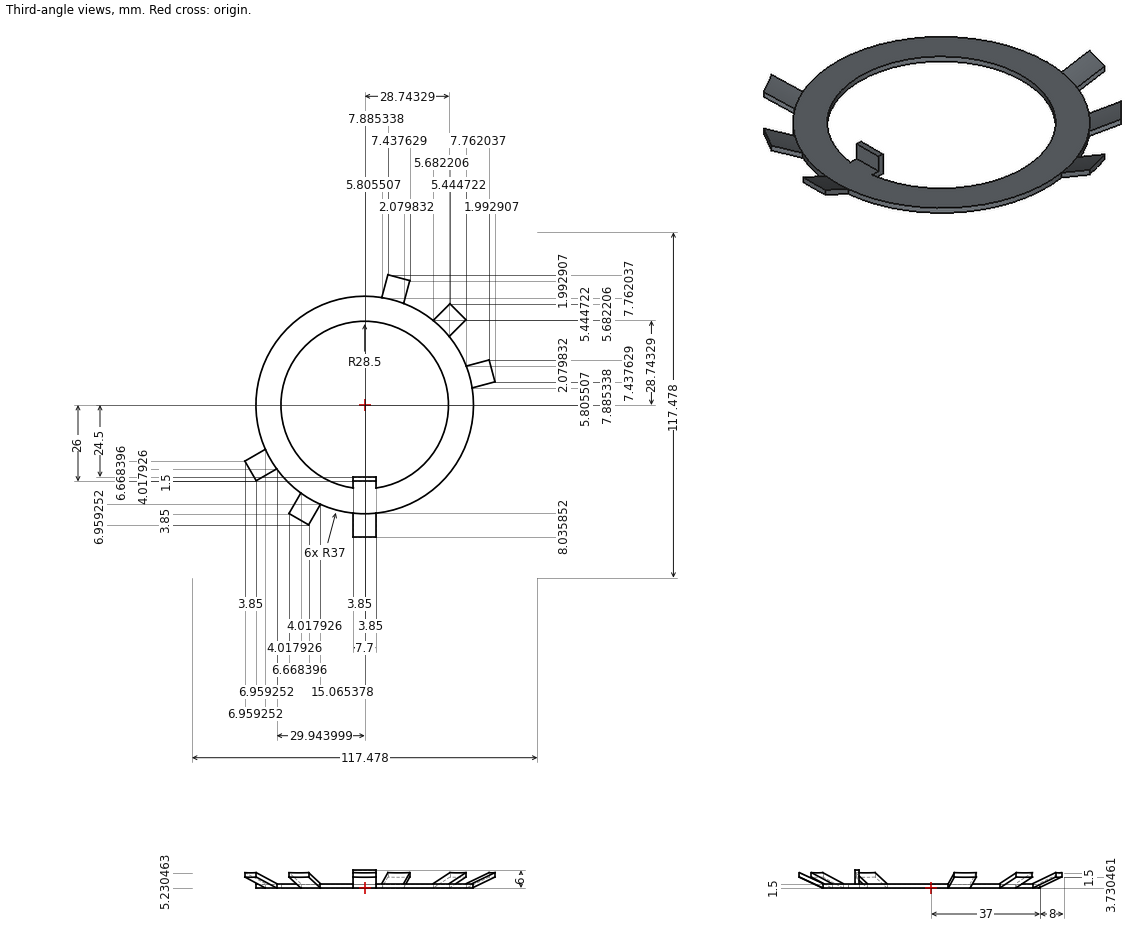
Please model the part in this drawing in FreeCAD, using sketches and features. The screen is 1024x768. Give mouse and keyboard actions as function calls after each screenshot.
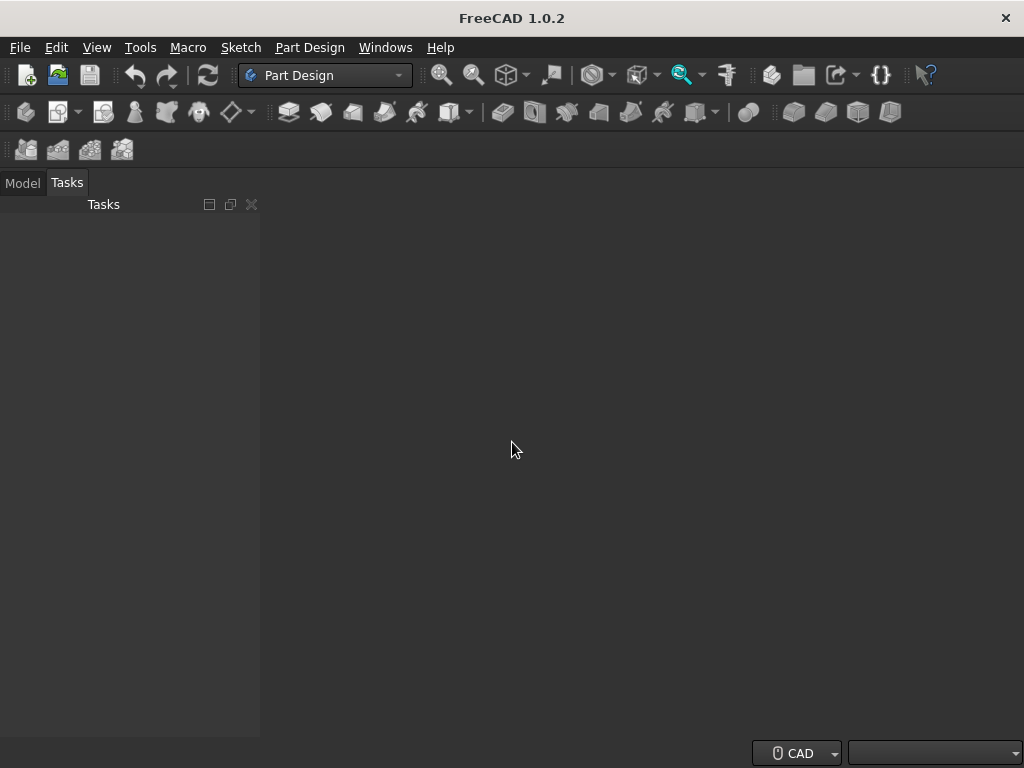
click(26, 76)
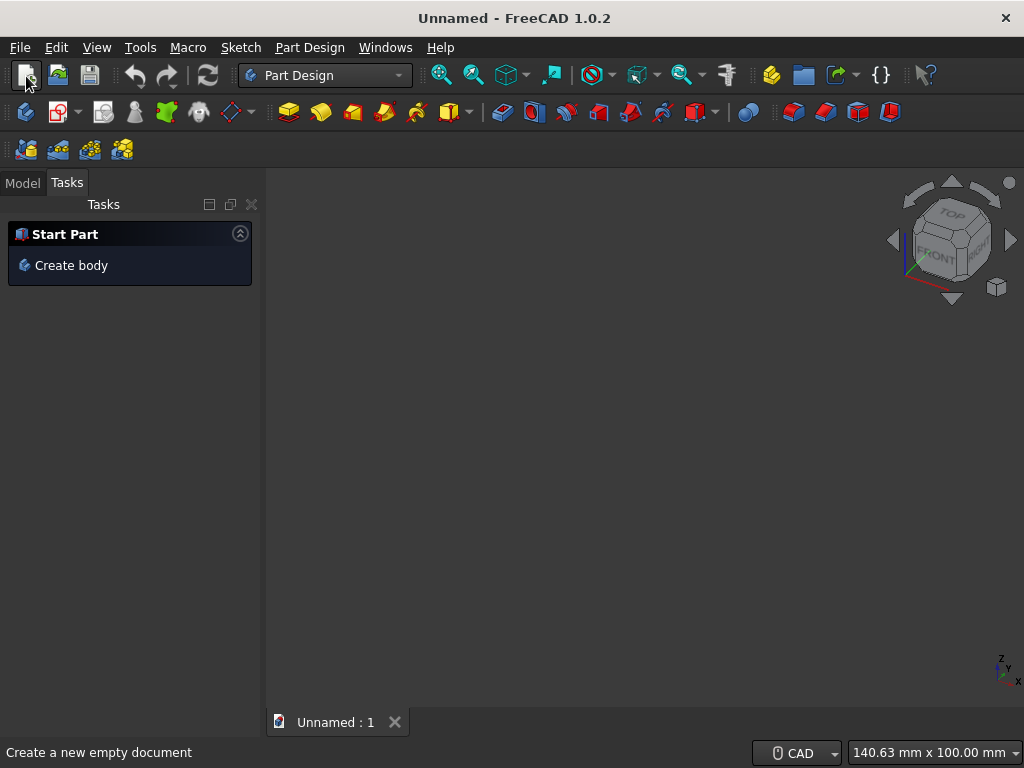
click(58, 112)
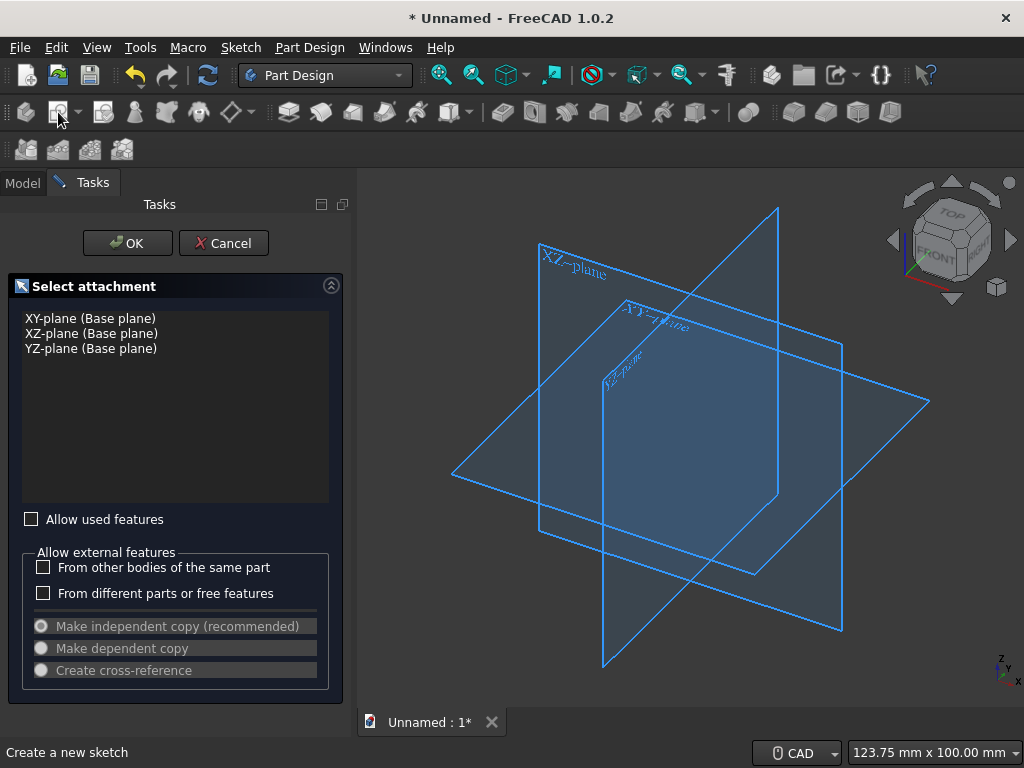
click(82, 348)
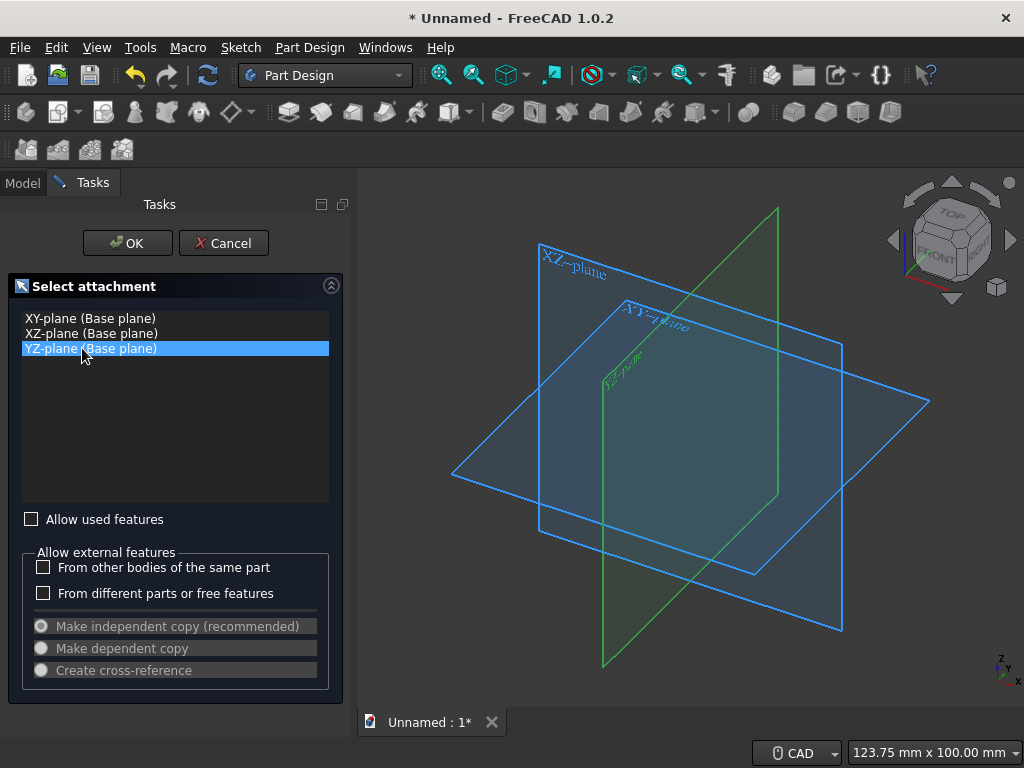
click(128, 243)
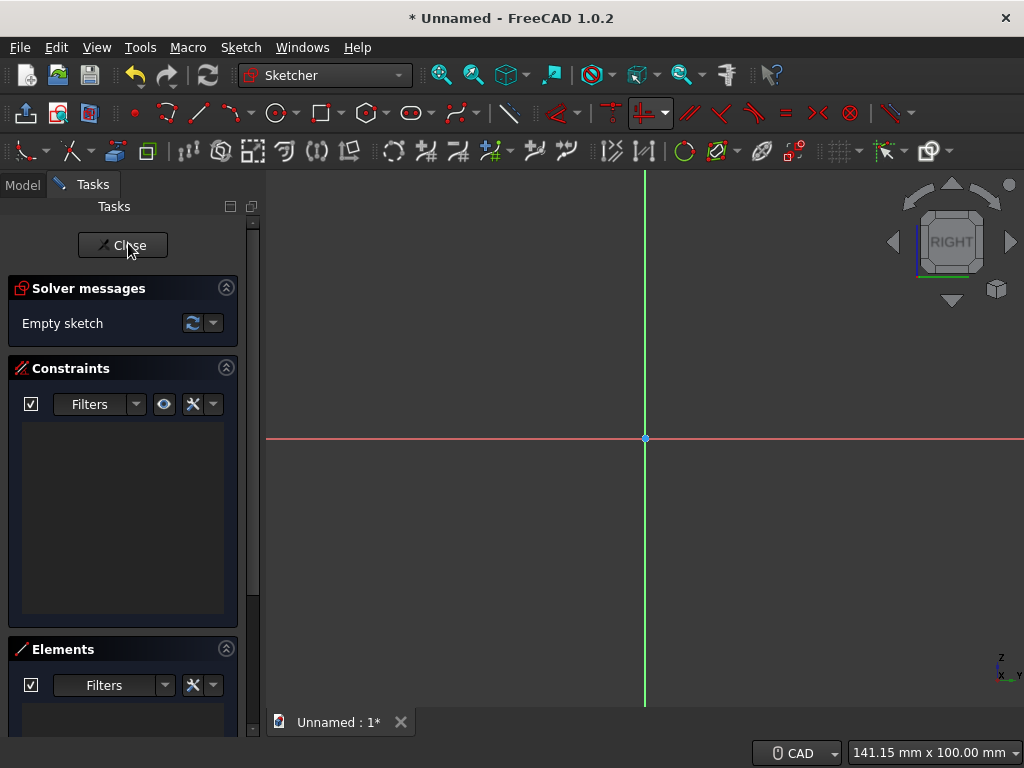
scroll(576, 438, down, 5)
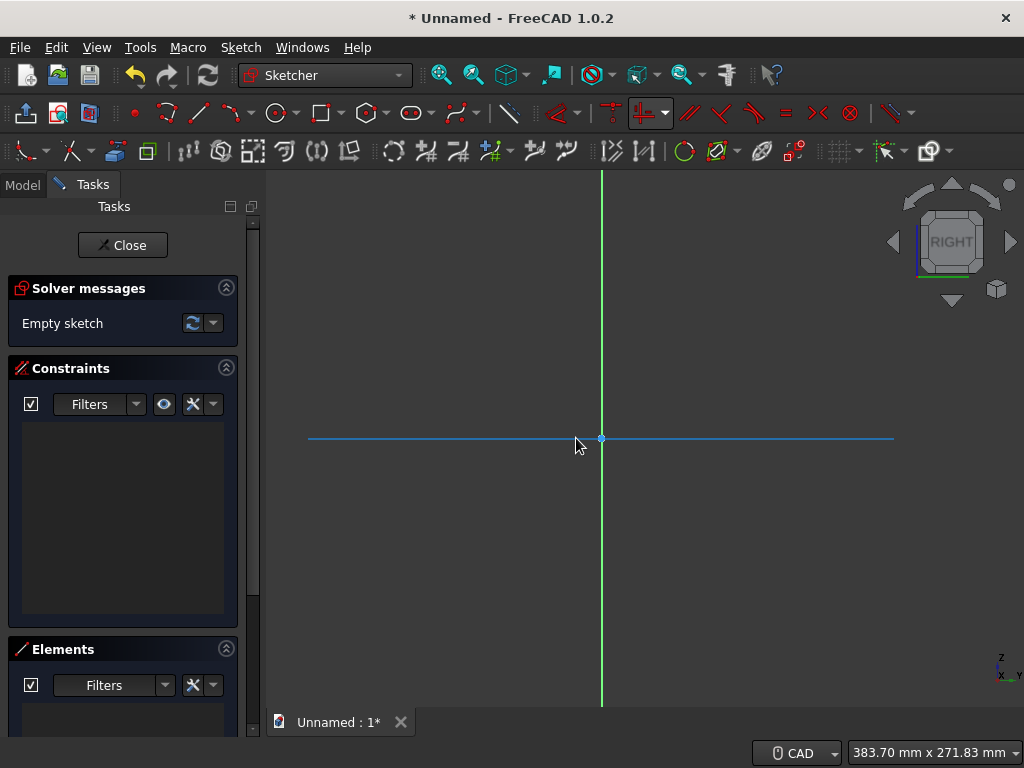
scroll(664, 432, up, 8)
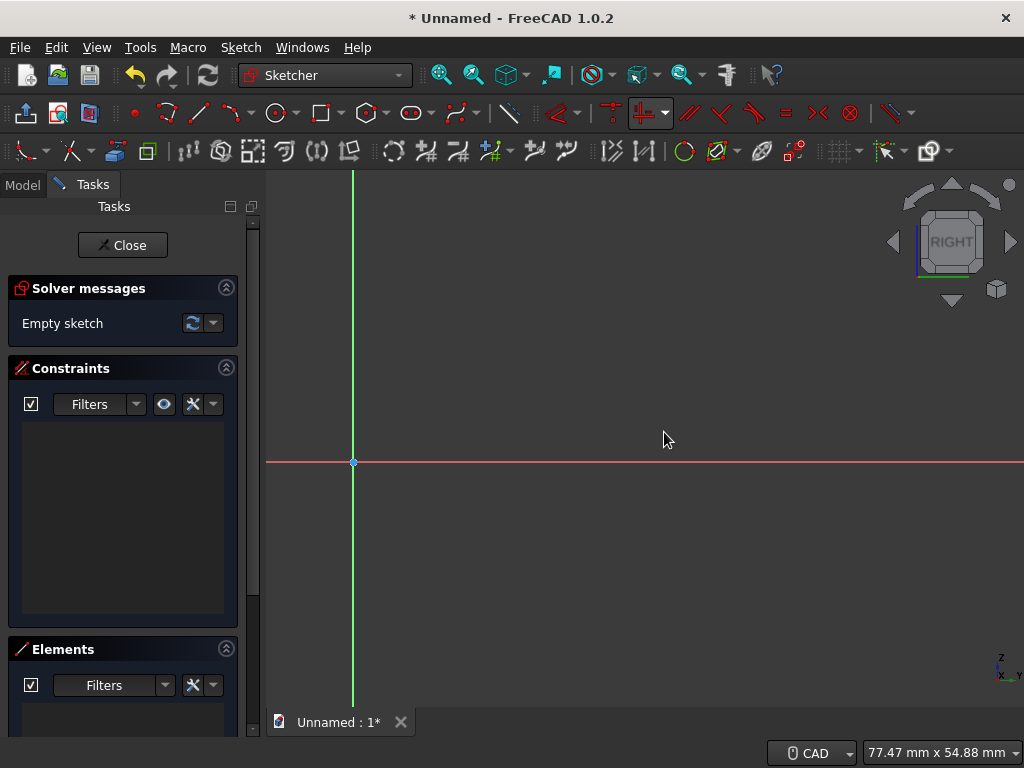
click(168, 114)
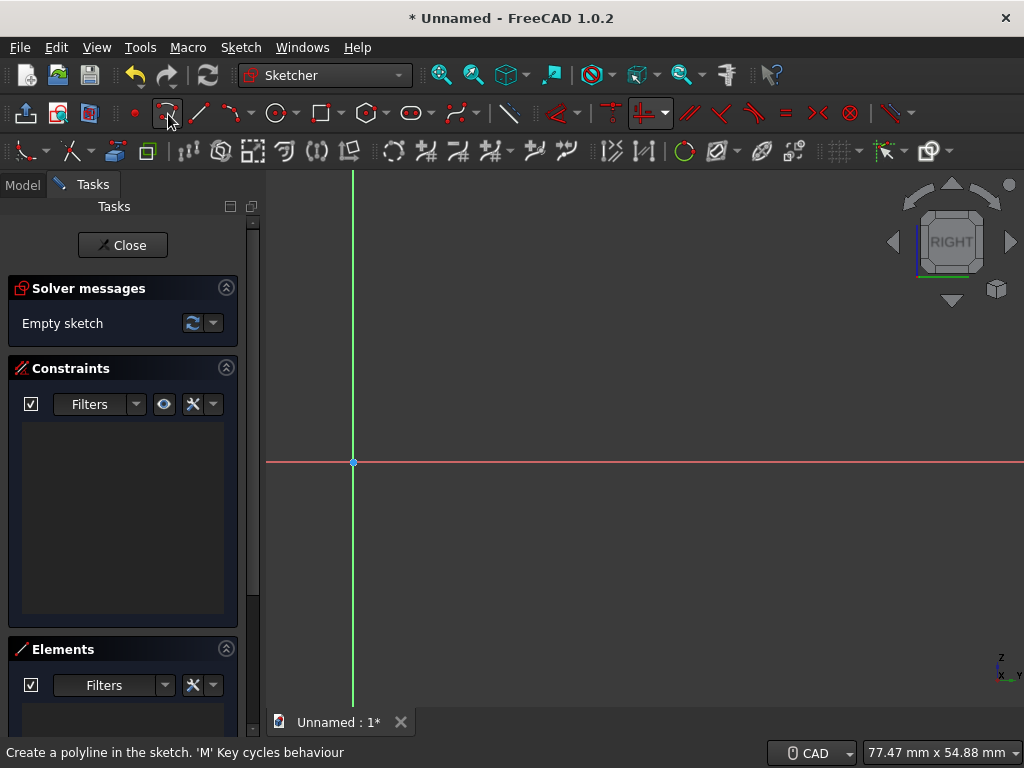
click(353, 462)
click(715, 453)
click(793, 426)
click(793, 411)
click(715, 448)
click(362, 448)
click(353, 462)
key(Escape)
key(Escape)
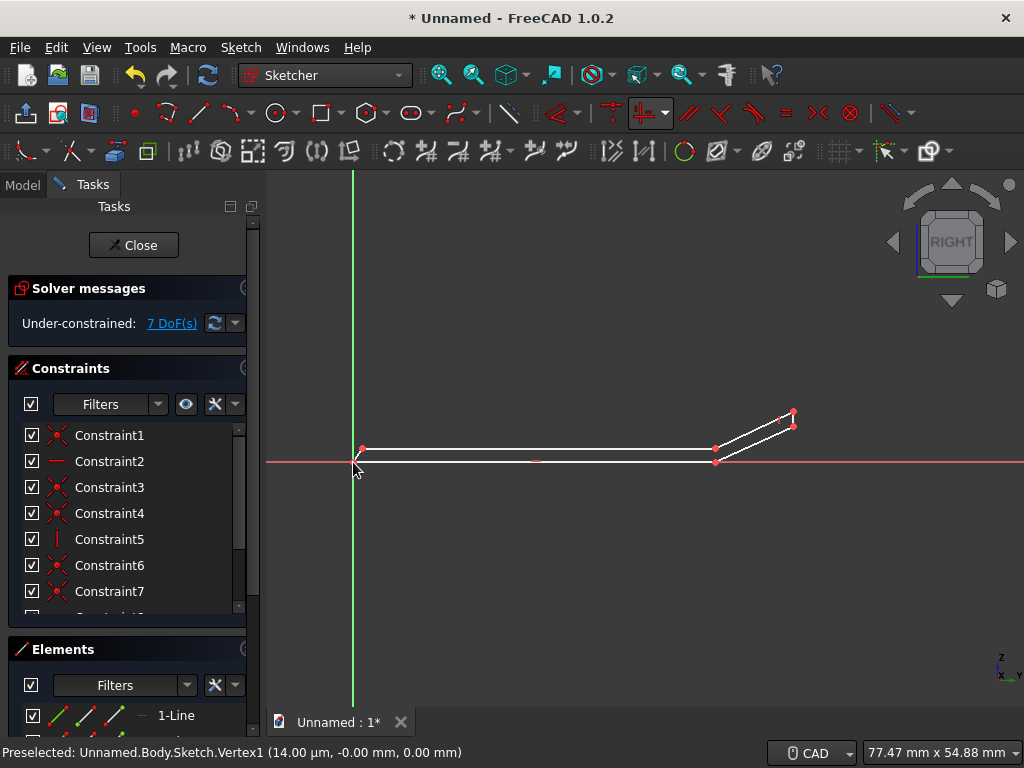
scroll(358, 454, up, 5)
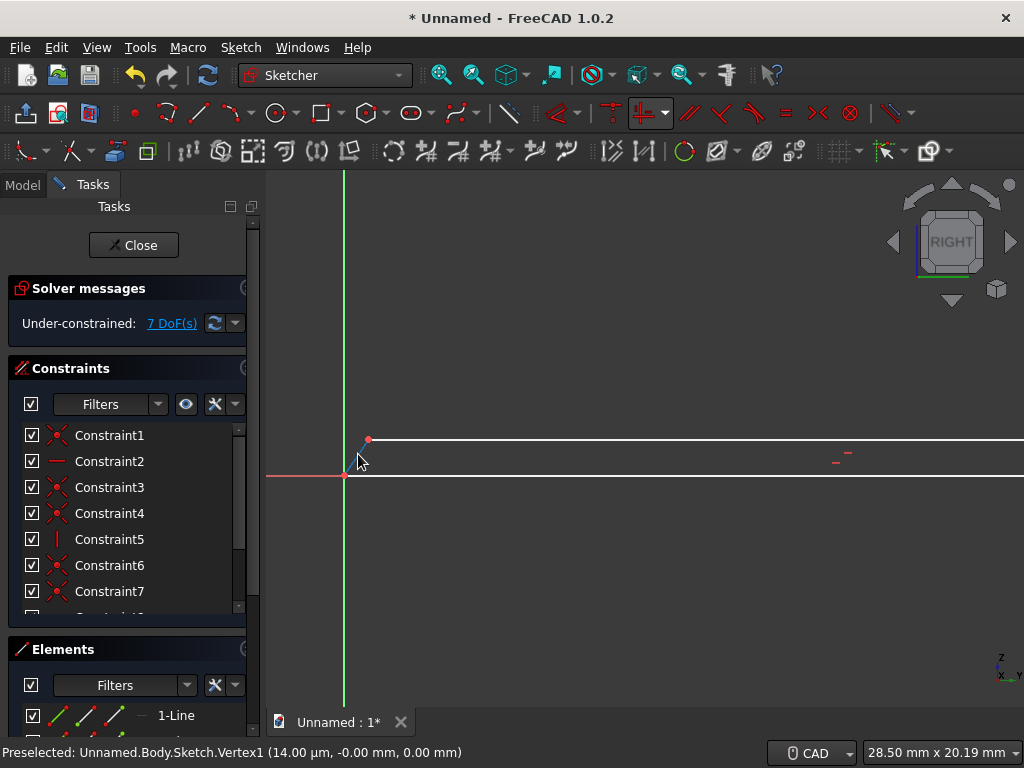
click(359, 454)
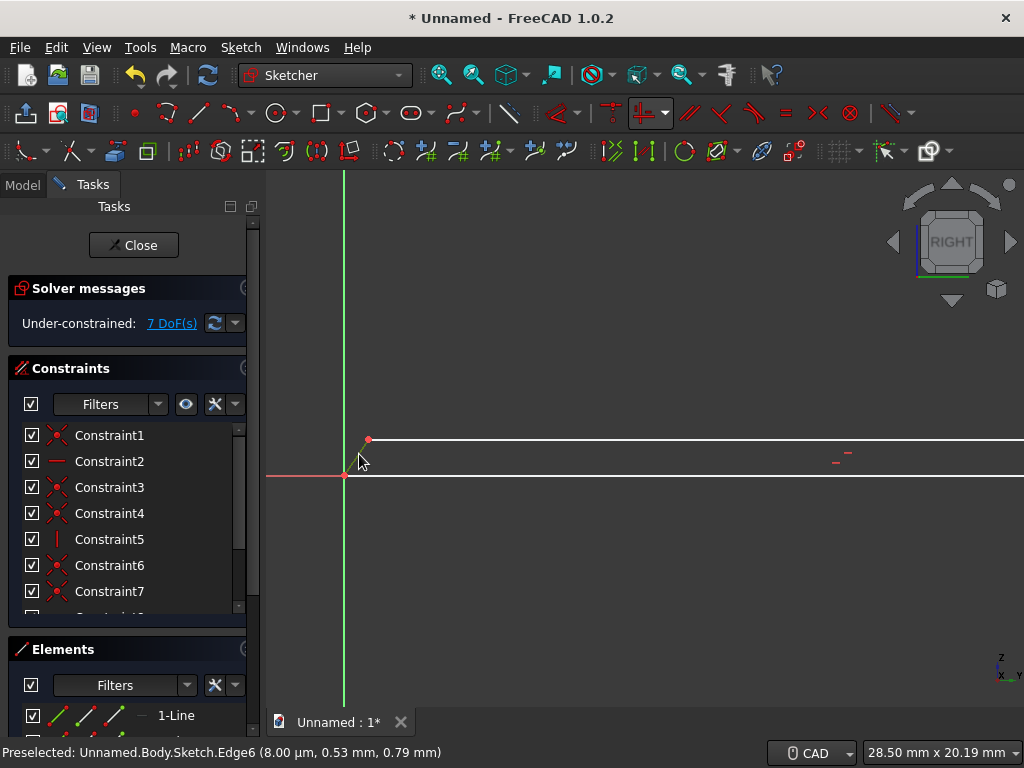
key(v)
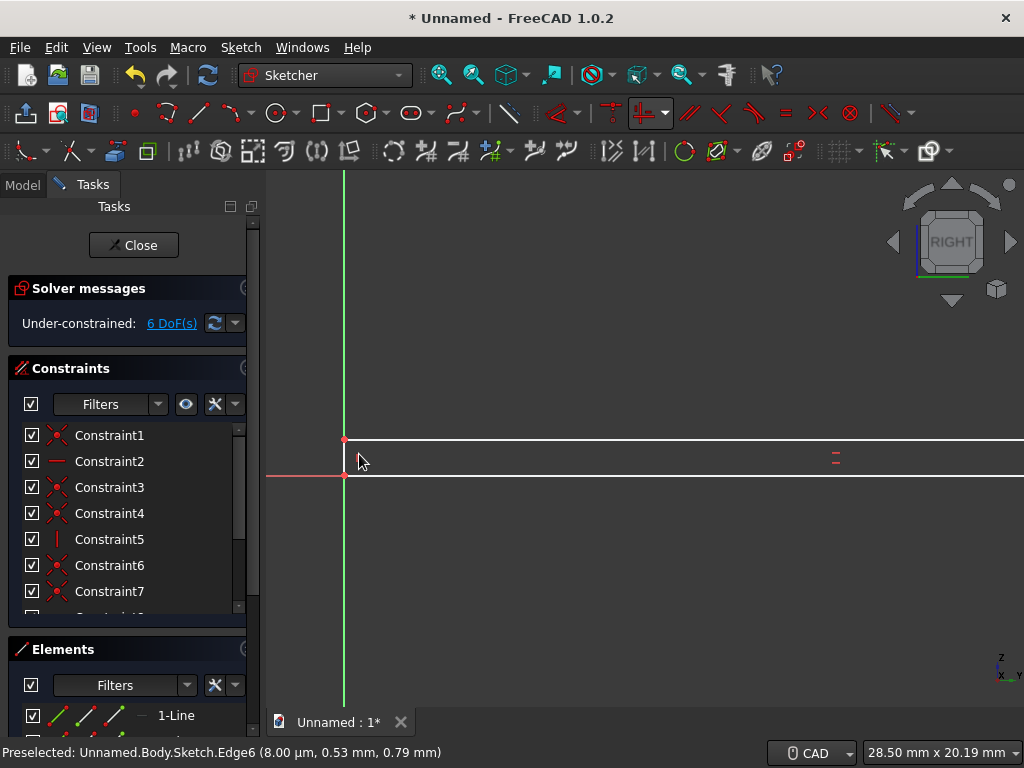
key(d)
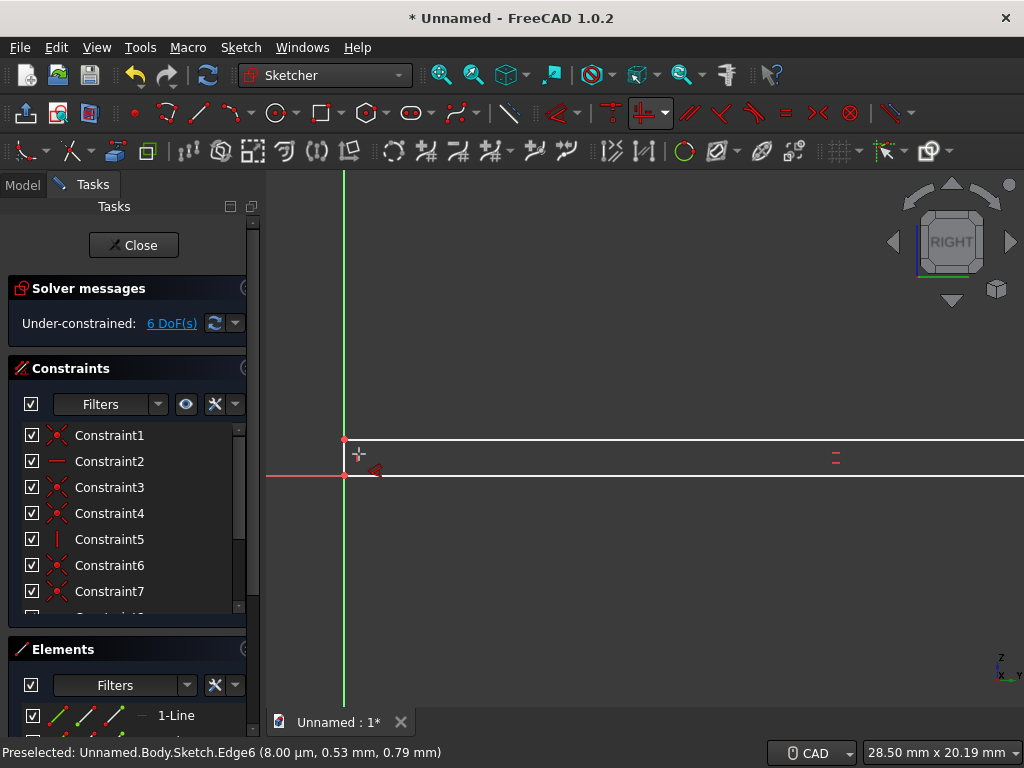
click(640, 476)
click(602, 510)